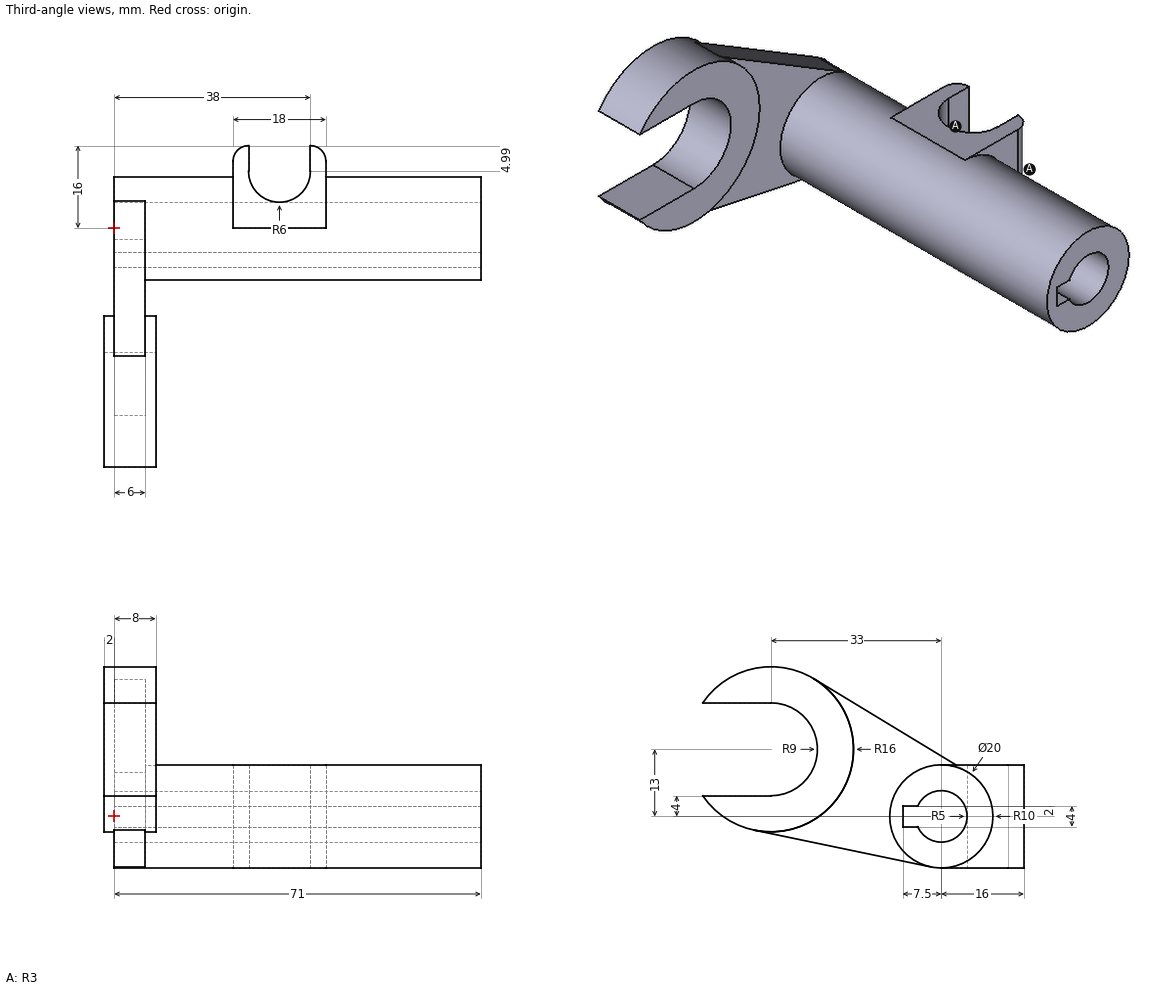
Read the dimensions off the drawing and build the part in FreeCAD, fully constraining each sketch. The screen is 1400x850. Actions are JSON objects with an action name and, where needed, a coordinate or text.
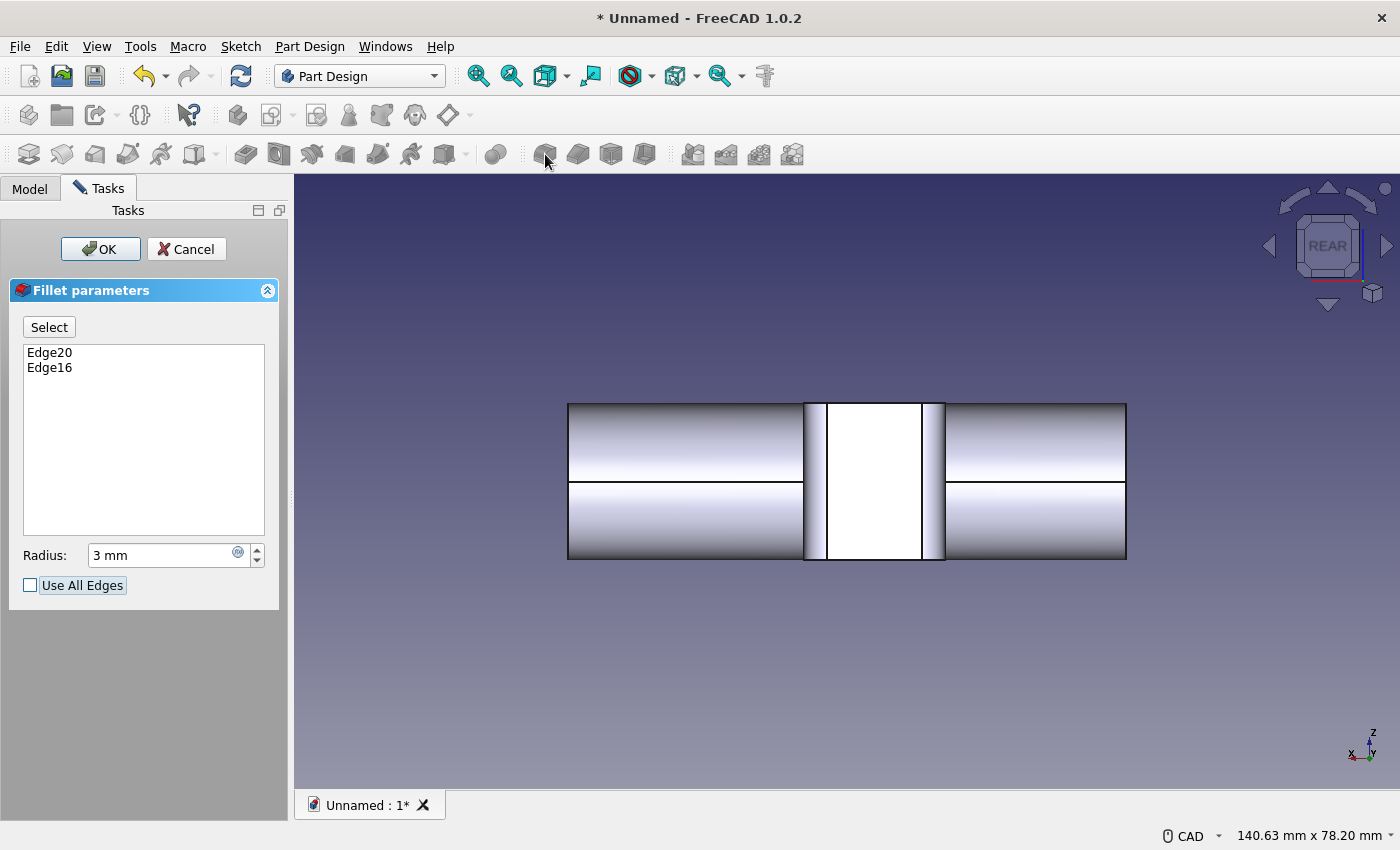
{"action": "left_click", "coordinate": [101, 249]}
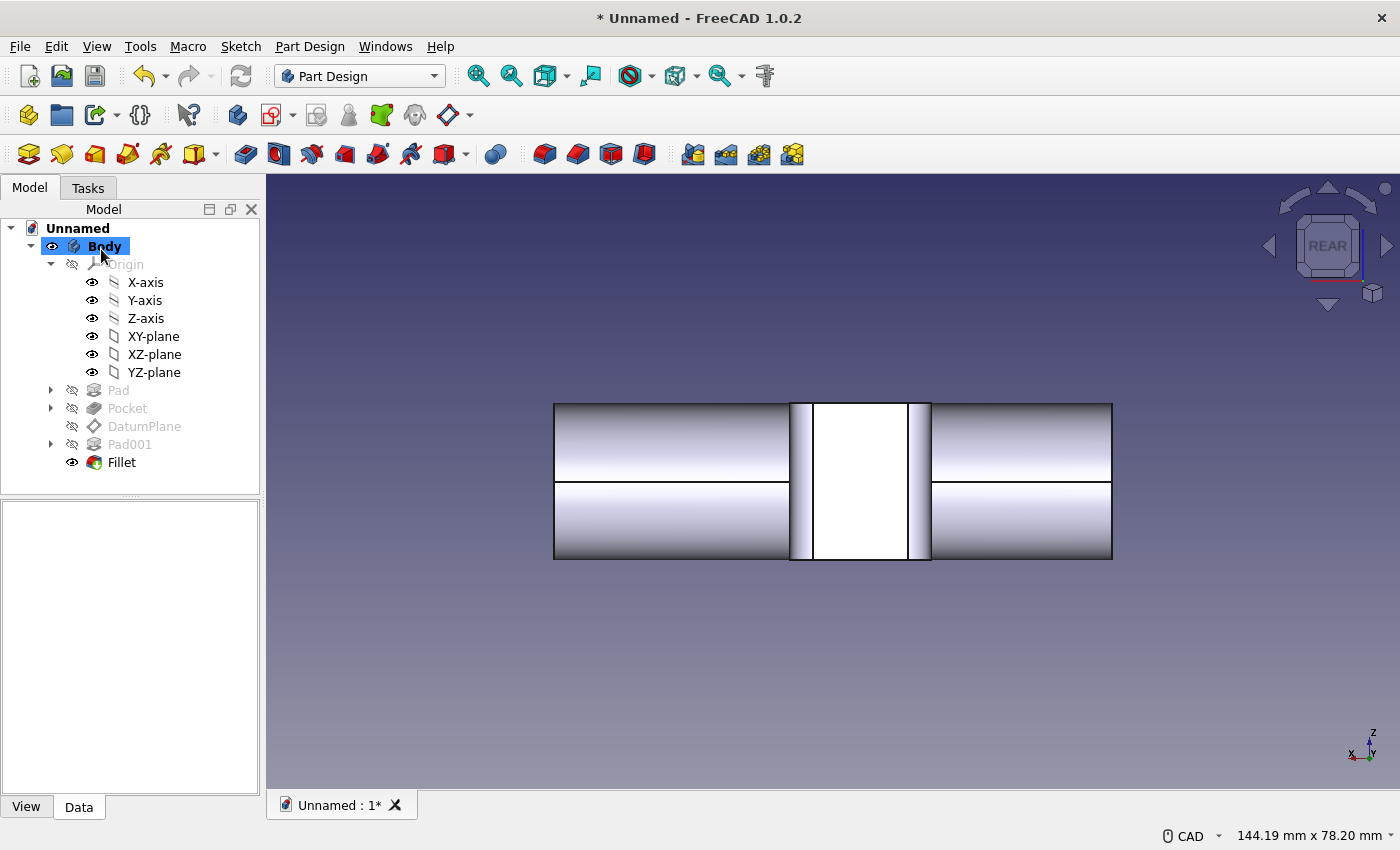
{"action": "left_click", "coordinate": [238, 116]}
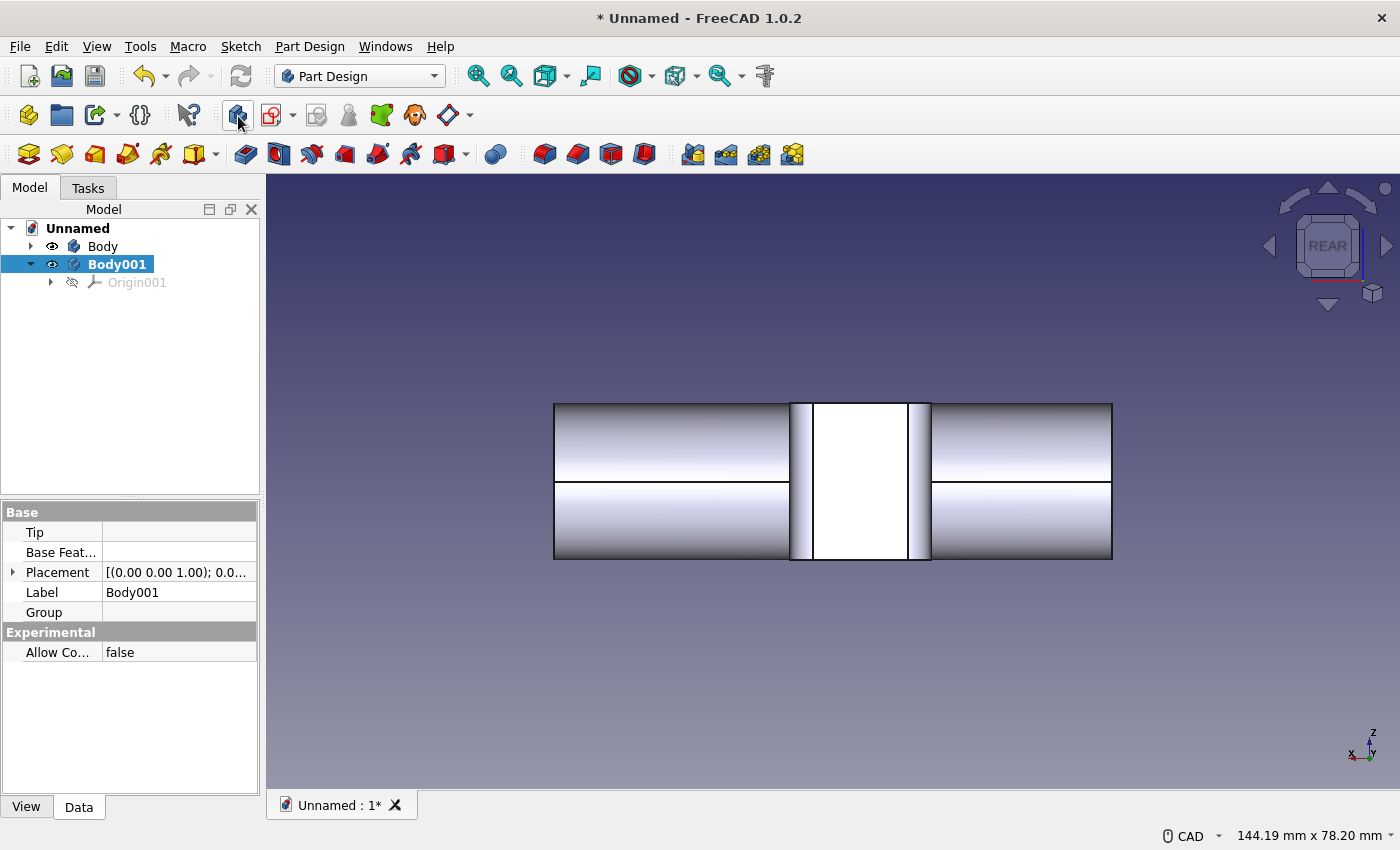
{"action": "left_click", "coordinate": [306, 749]}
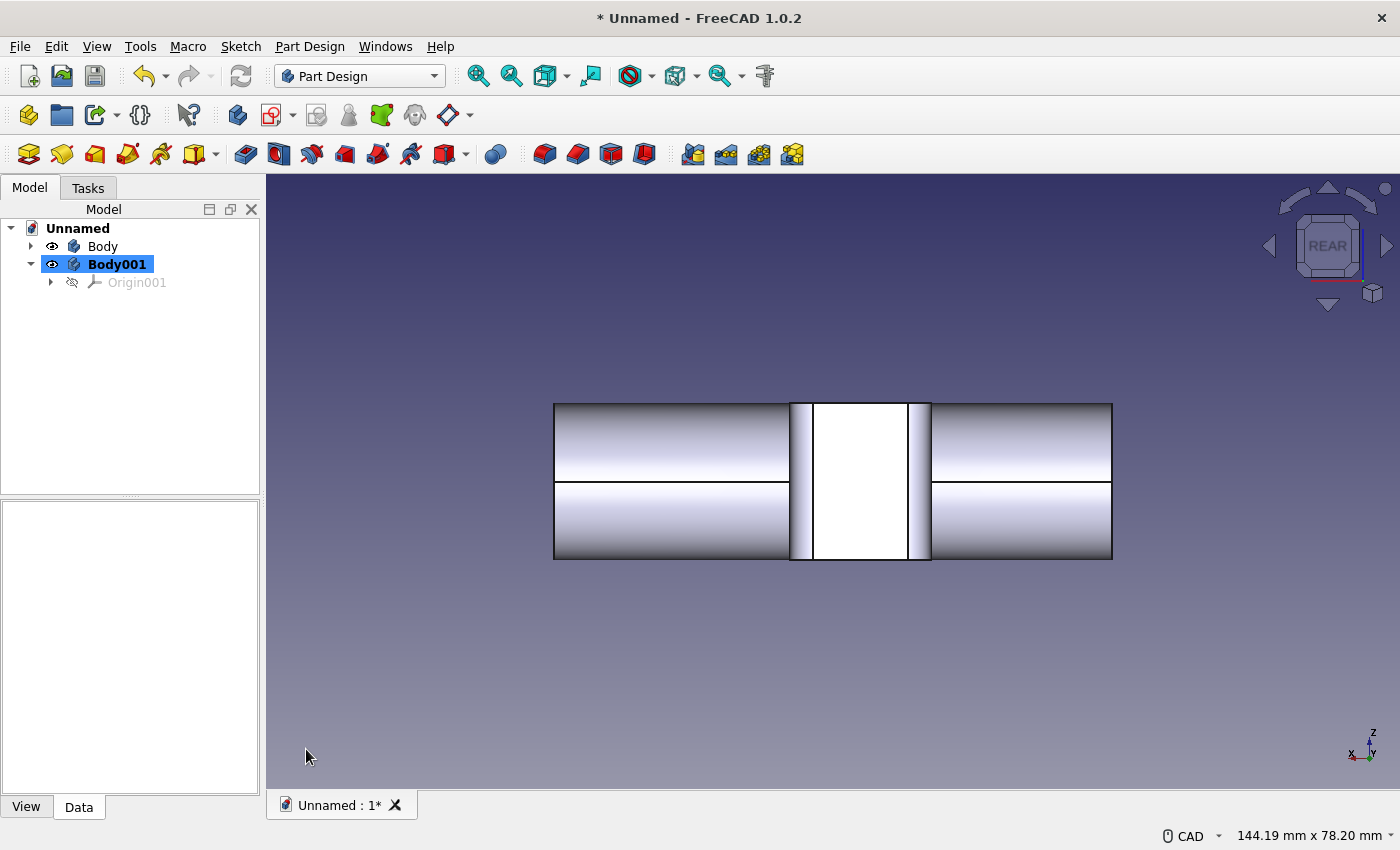
{"action": "left_click", "coordinate": [270, 116]}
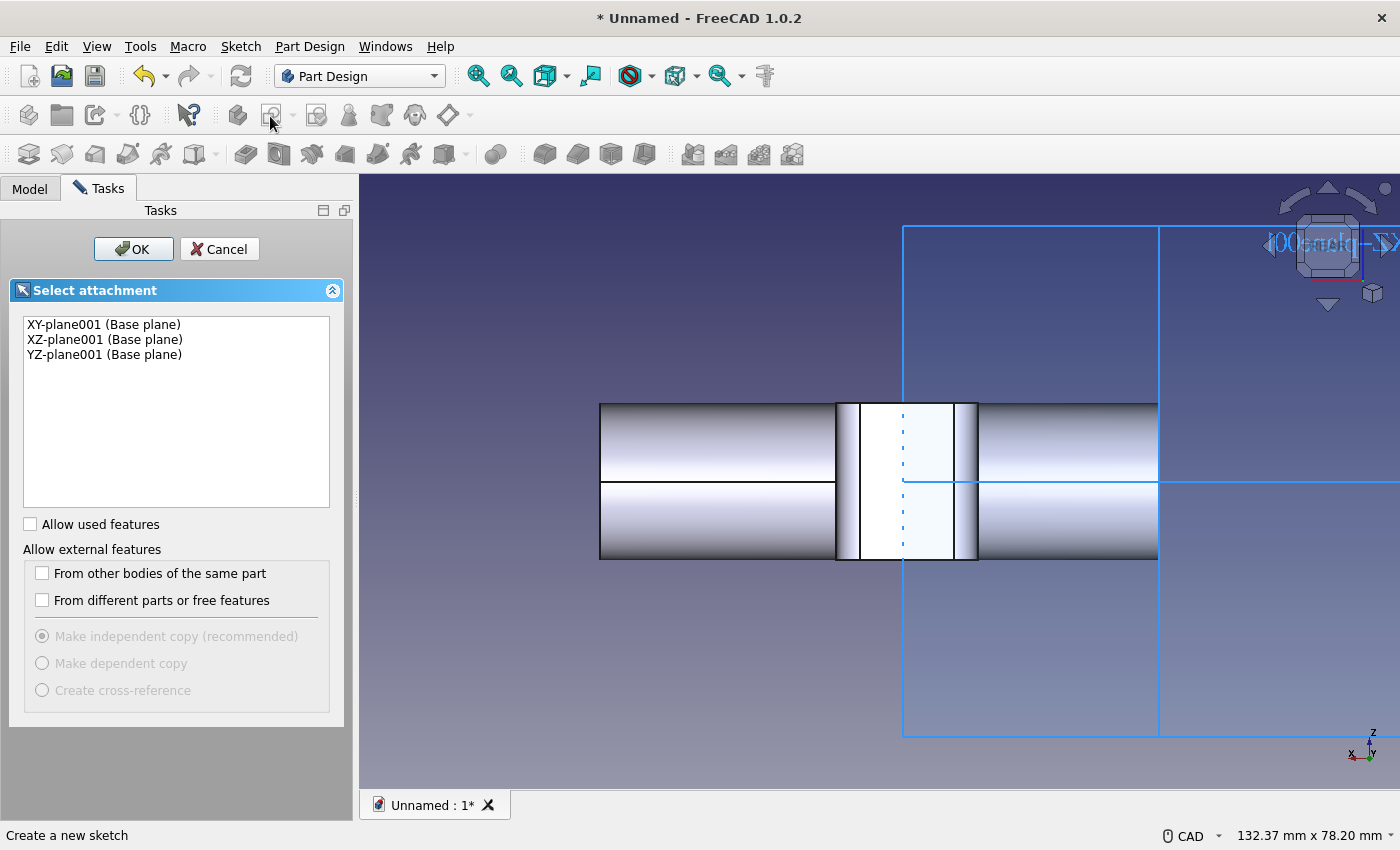
{"action": "left_click", "coordinate": [84, 354]}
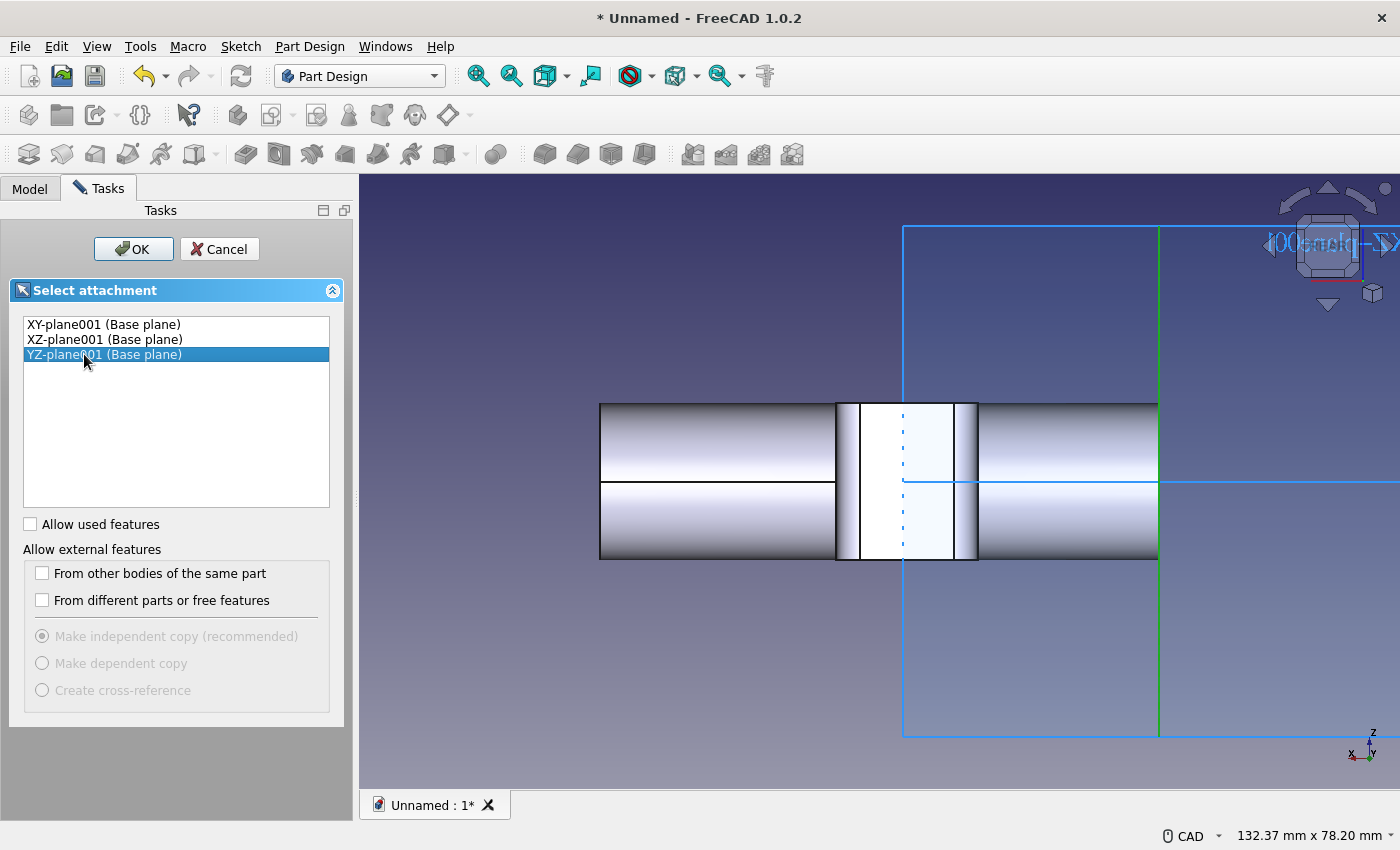
{"action": "left_click", "coordinate": [134, 249]}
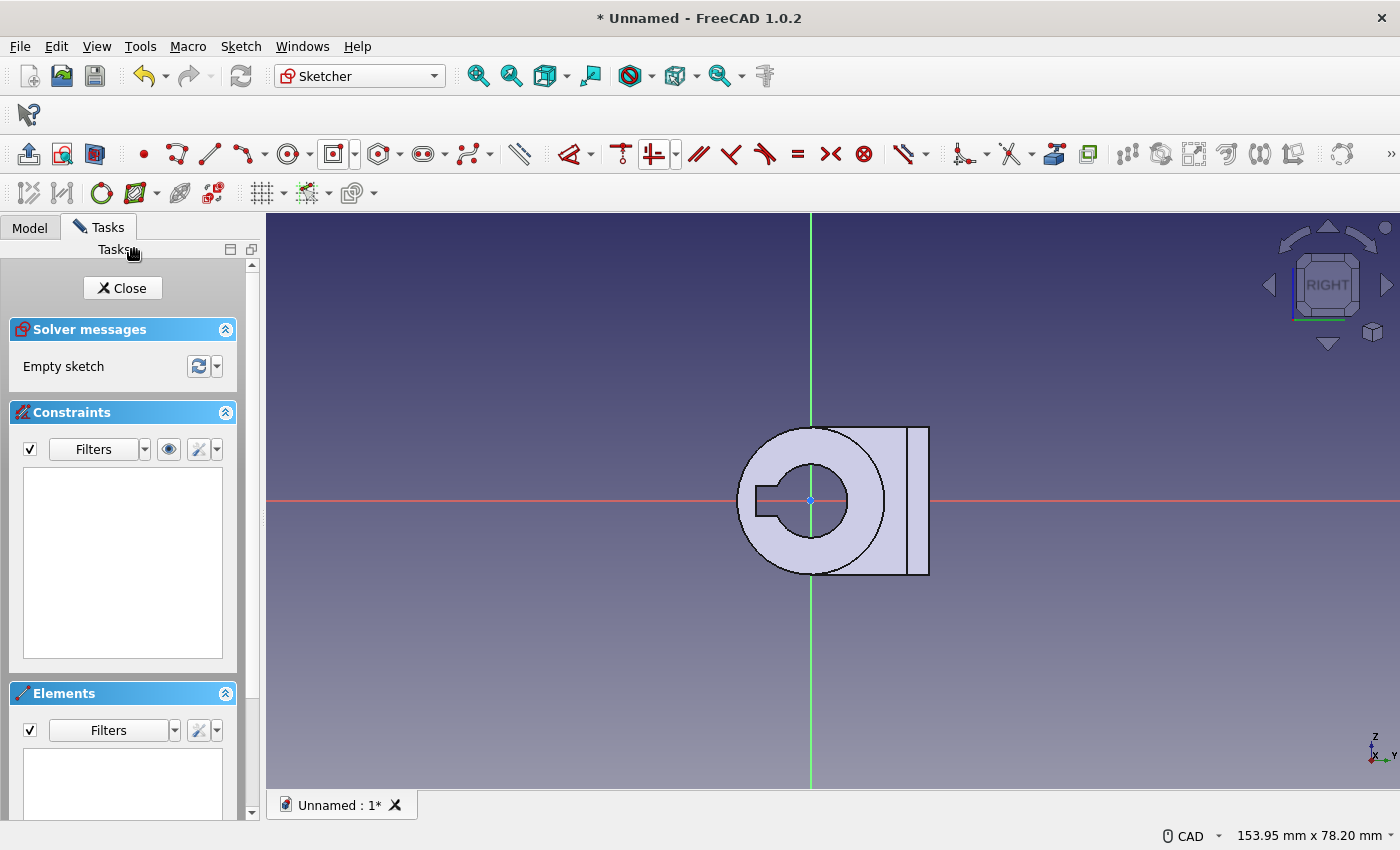
{"action": "scroll", "coordinate": [490, 321], "scroll_direction": "up", "scroll_amount": 3}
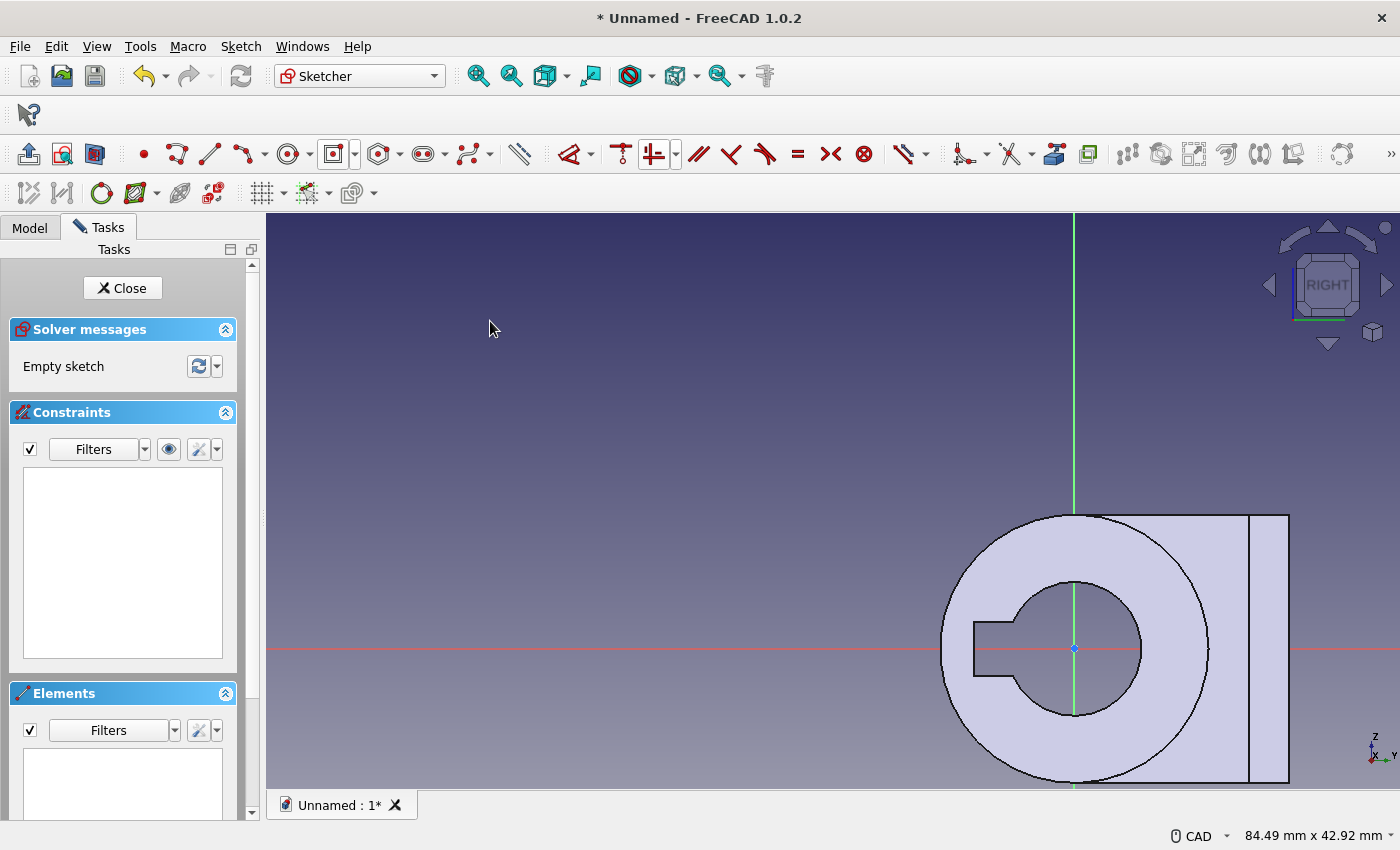
{"action": "key", "text": "g l"}